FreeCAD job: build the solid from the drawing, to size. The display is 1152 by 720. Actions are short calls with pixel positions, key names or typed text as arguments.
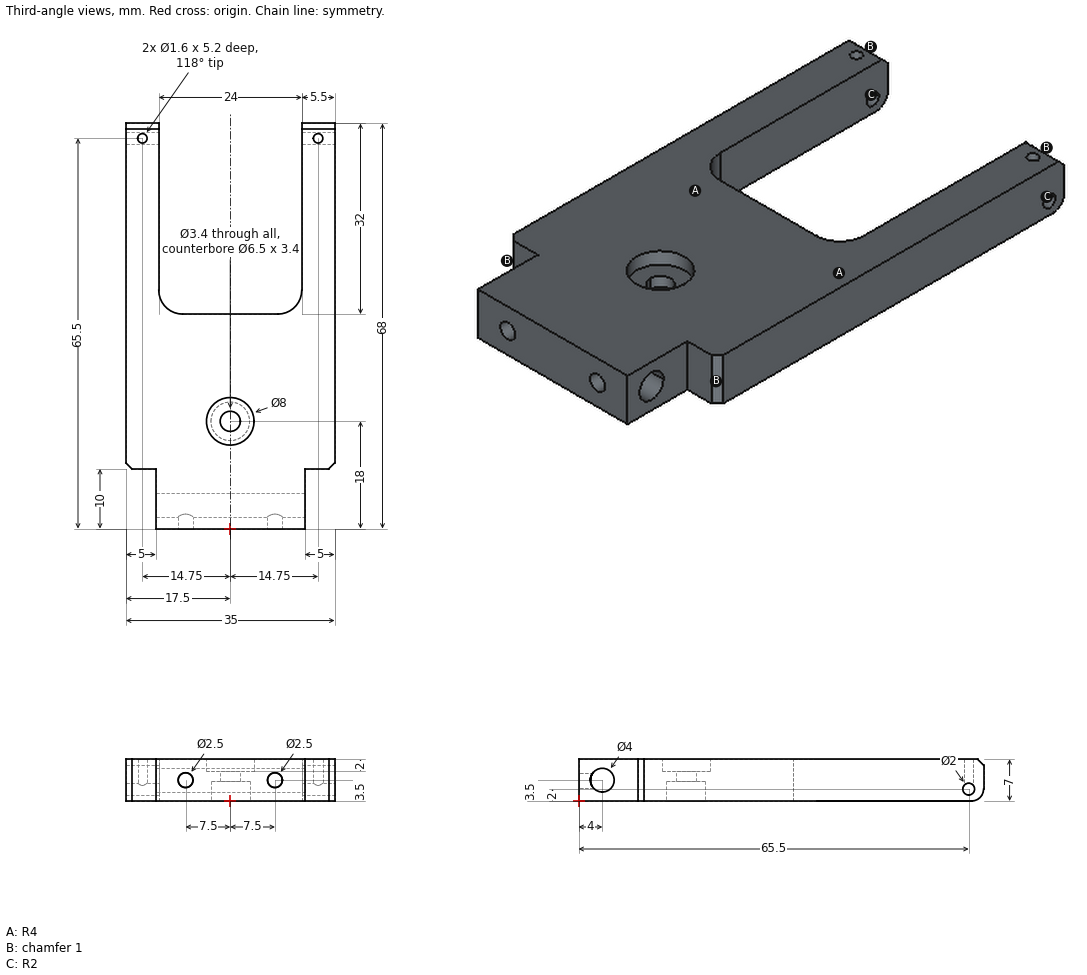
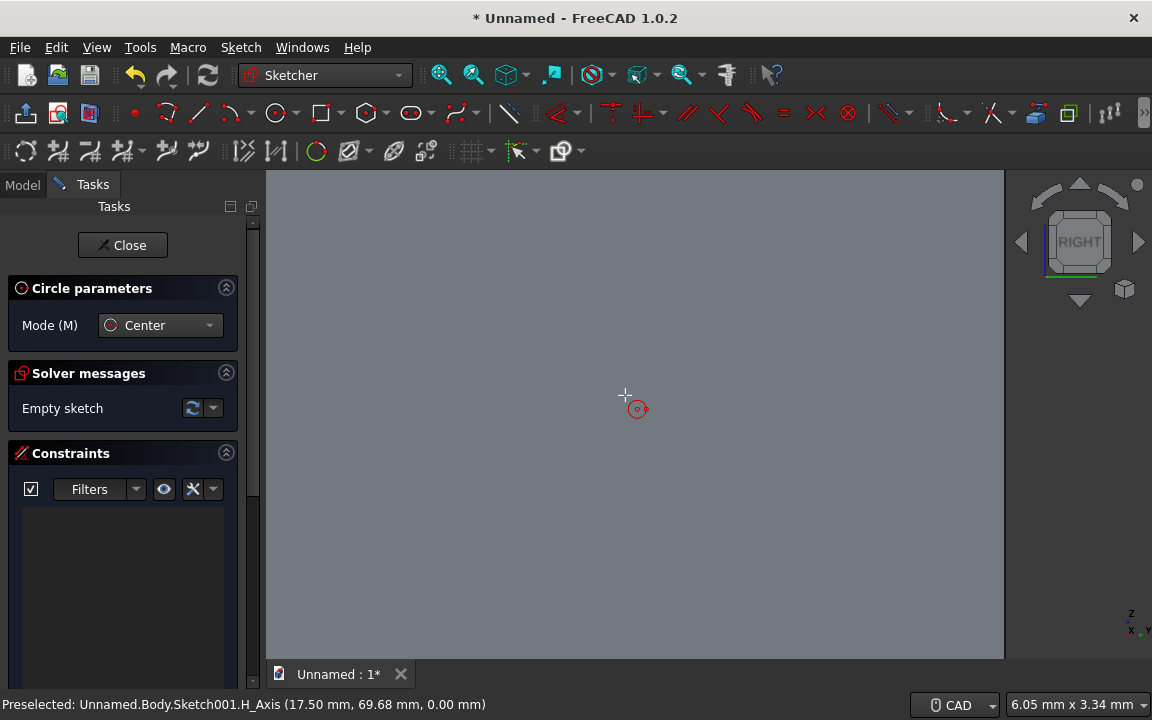
click(639, 412)
move(742, 309)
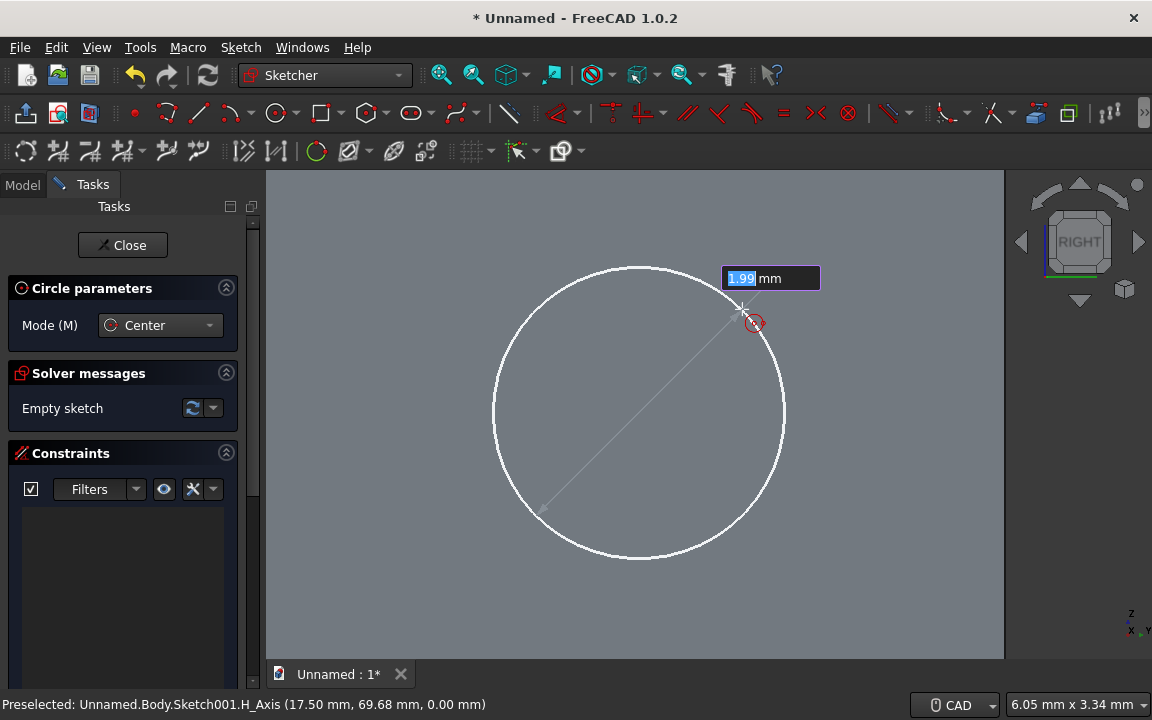
text(2)
key(Return)
key(Escape)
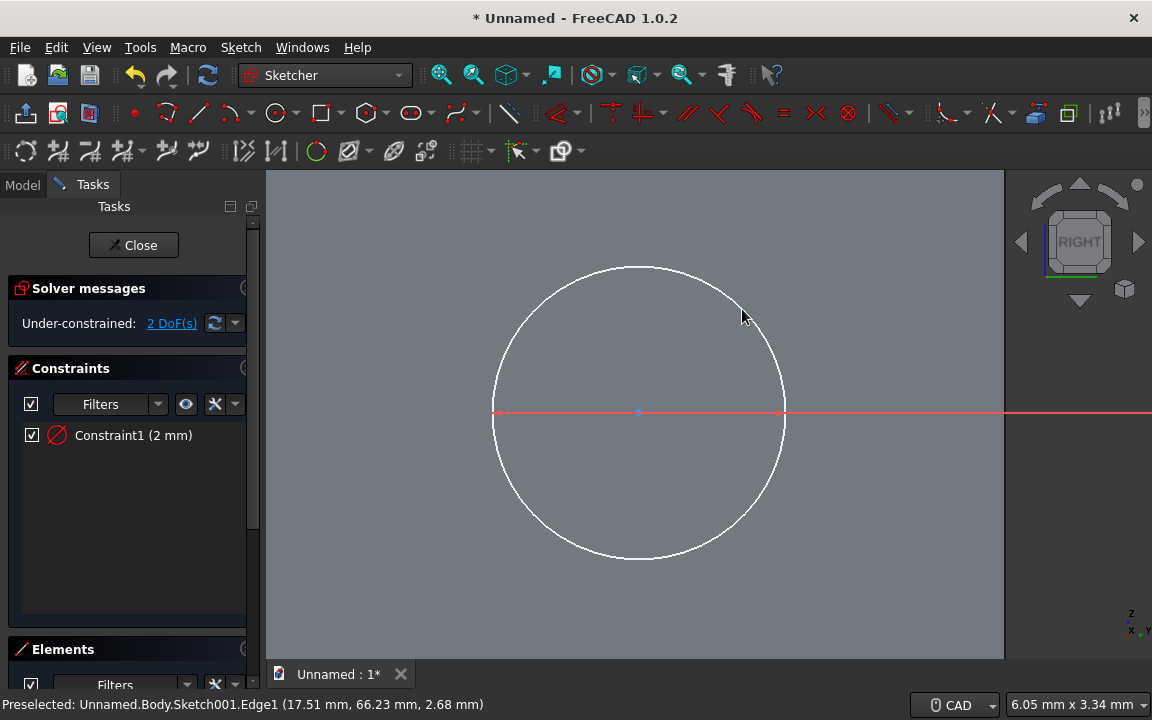
key(d)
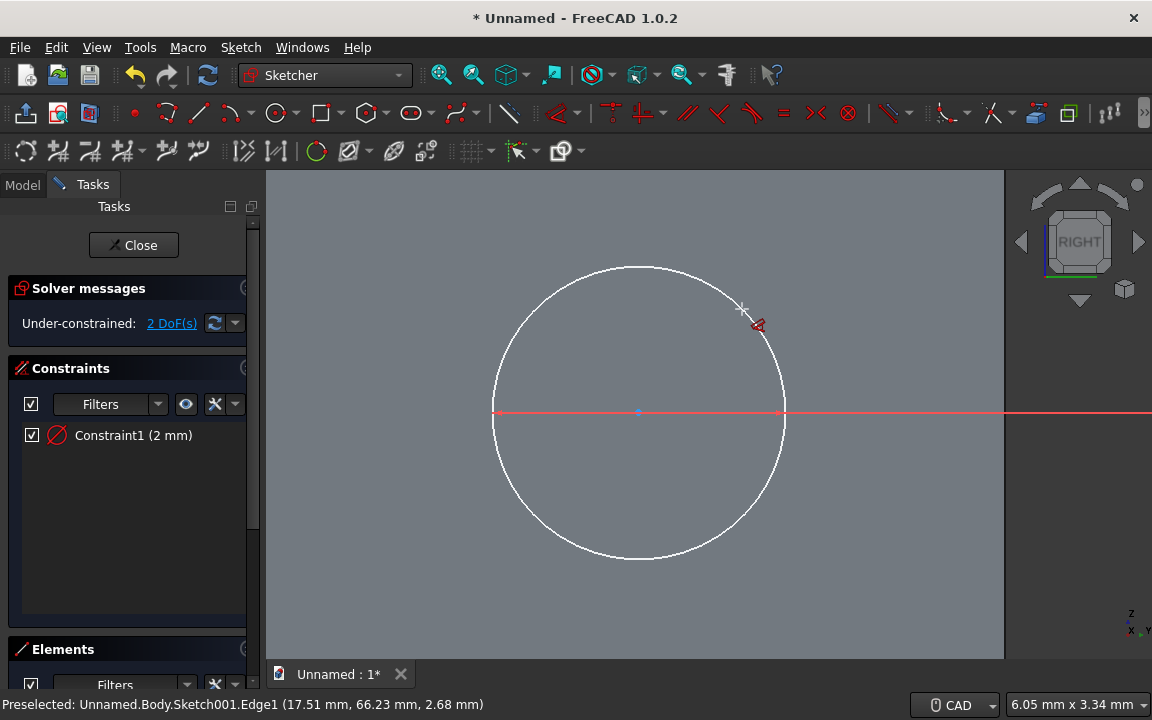
click(639, 413)
click(673, 522)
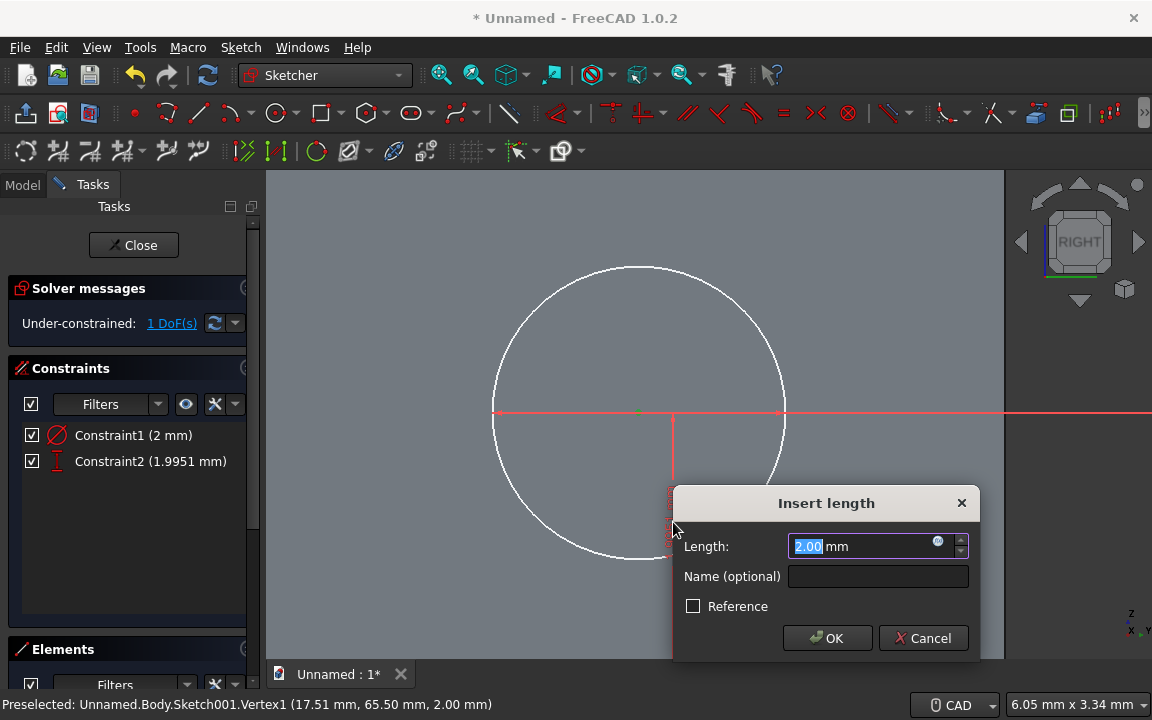
text(2)
key(Return)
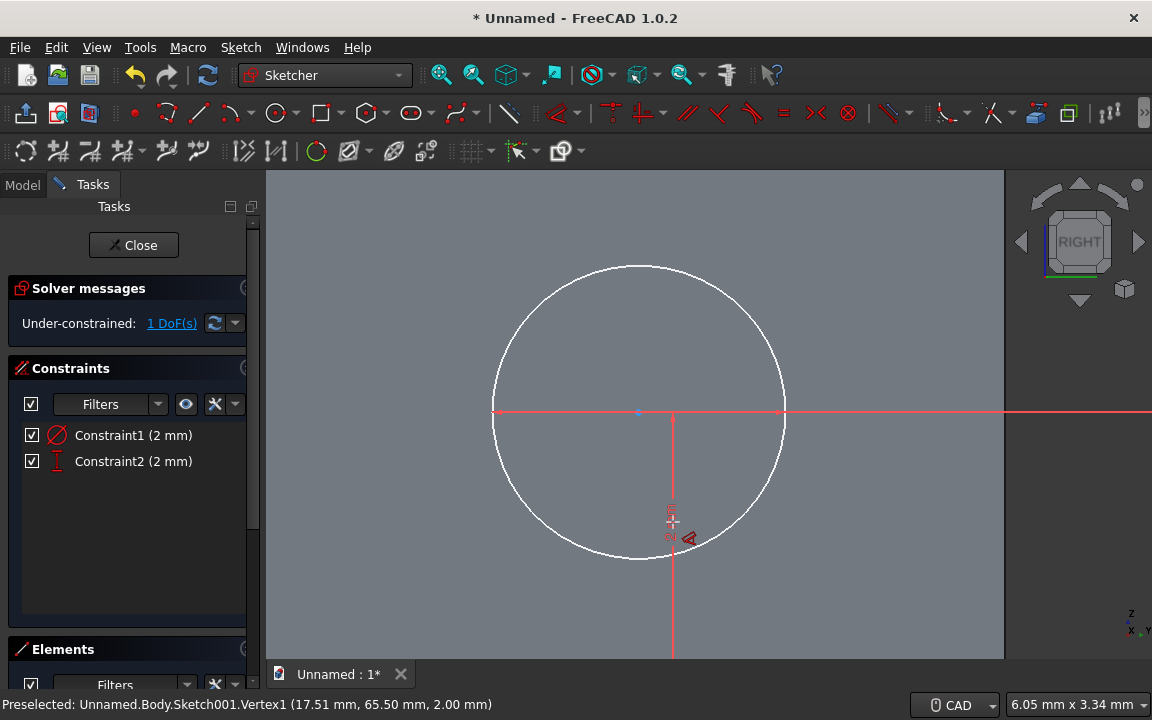
click(639, 412)
click(466, 378)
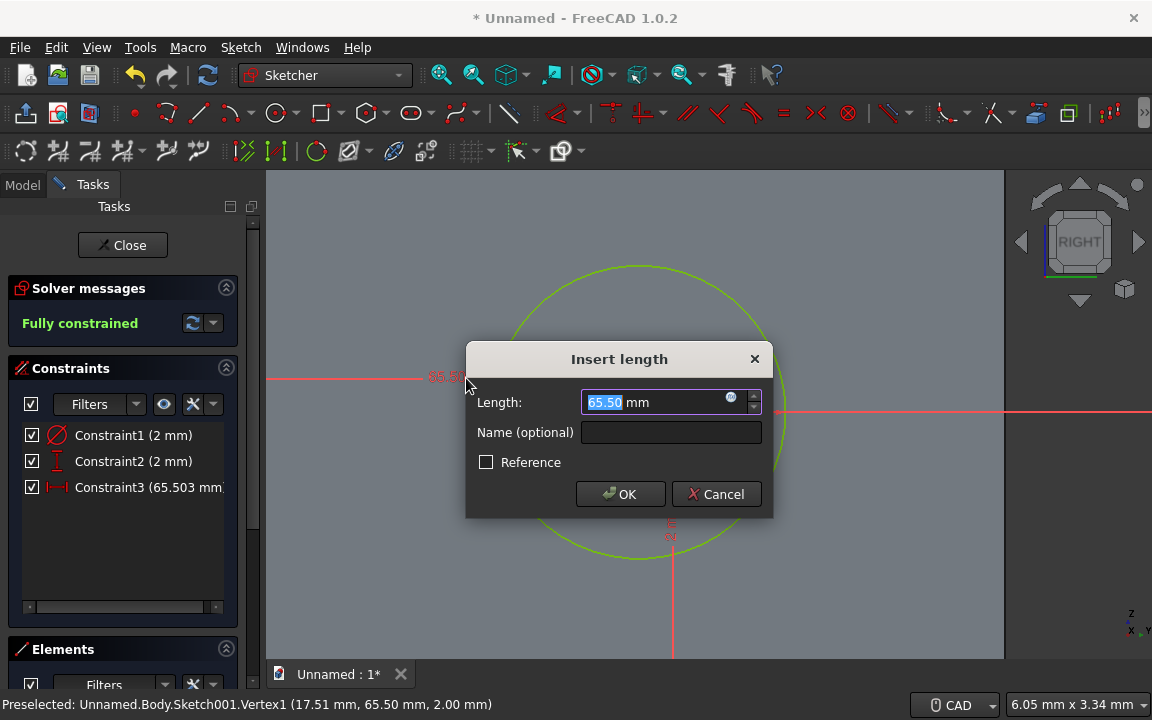
text(65.5)
key(Return)
key(Escape)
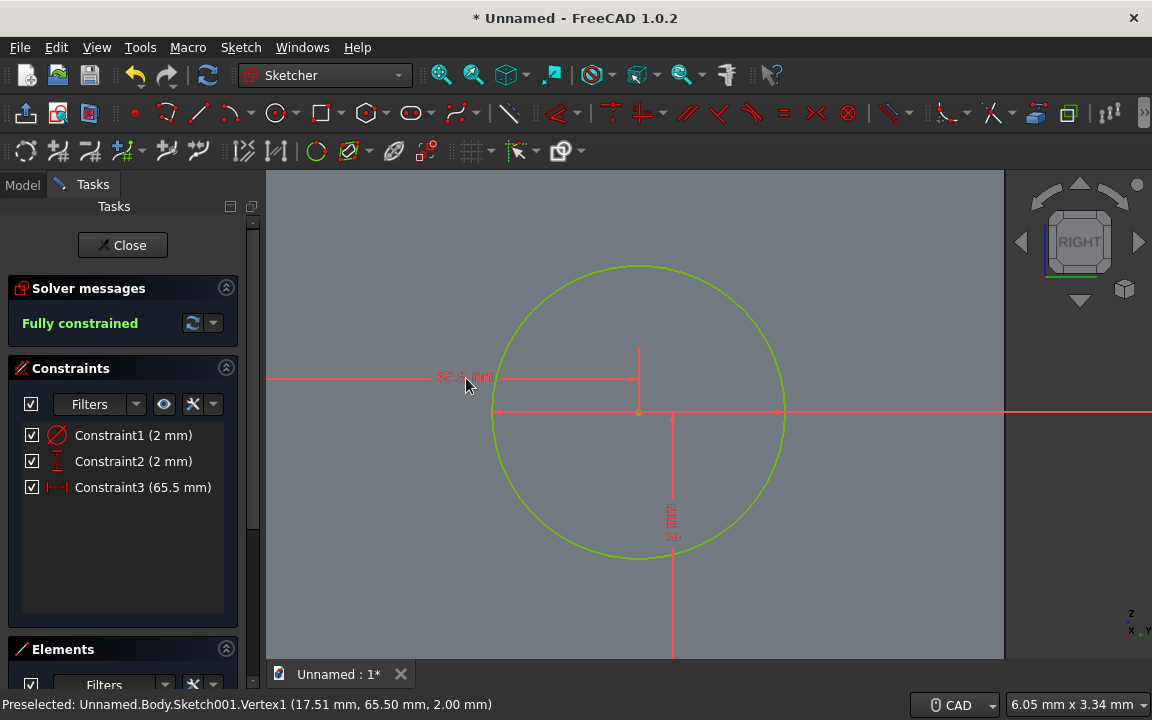
click(123, 245)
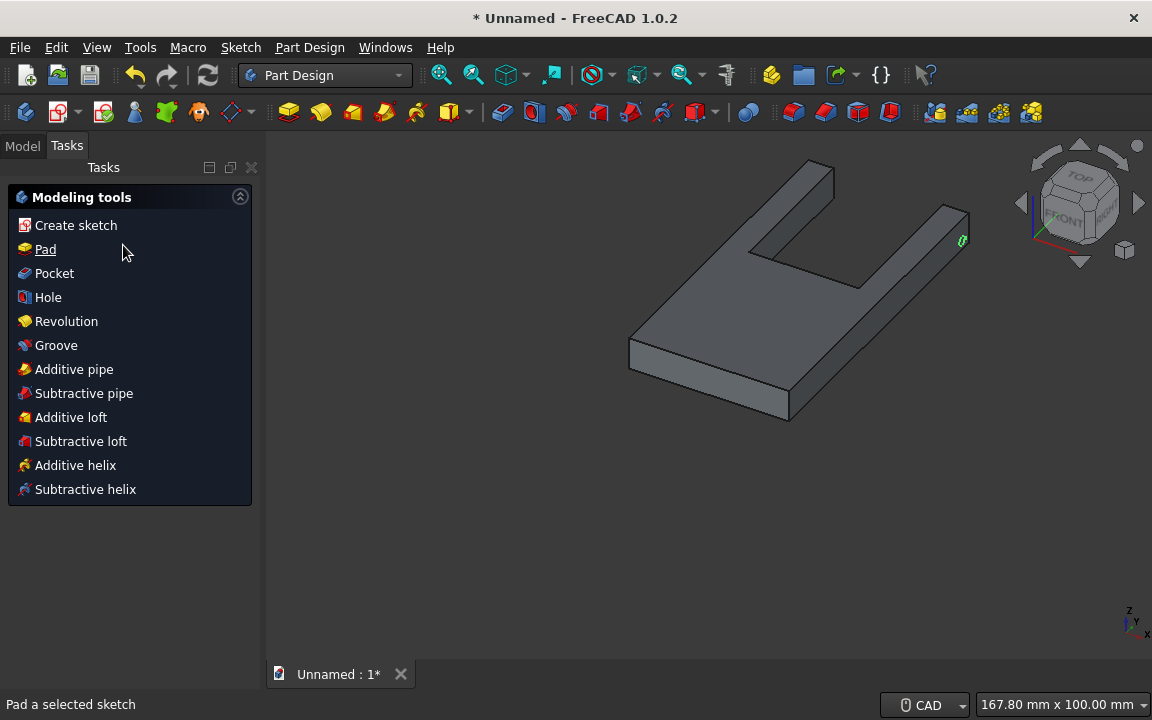
click(504, 112)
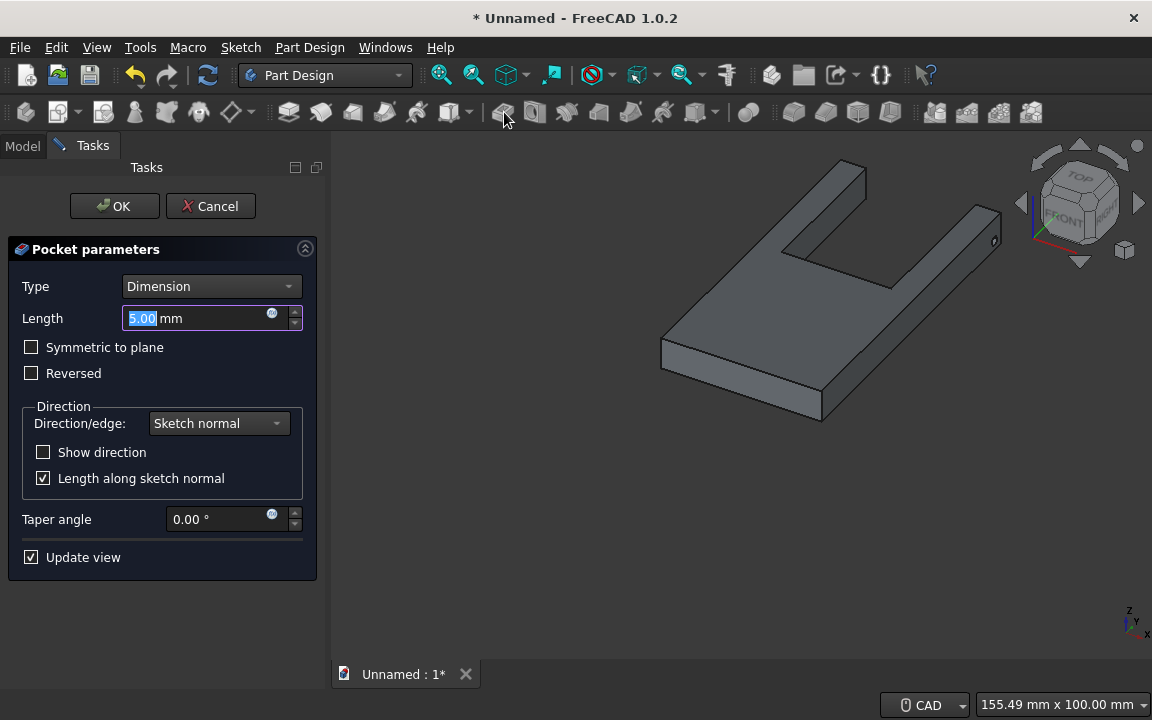
click(212, 286)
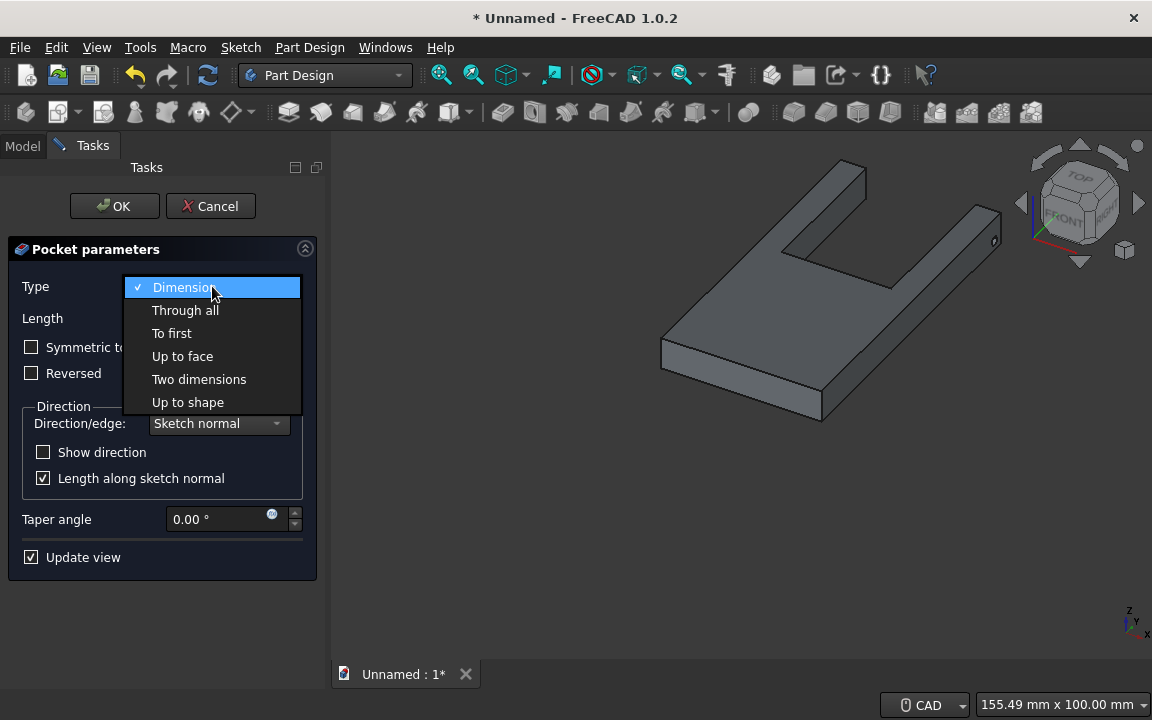
click(212, 310)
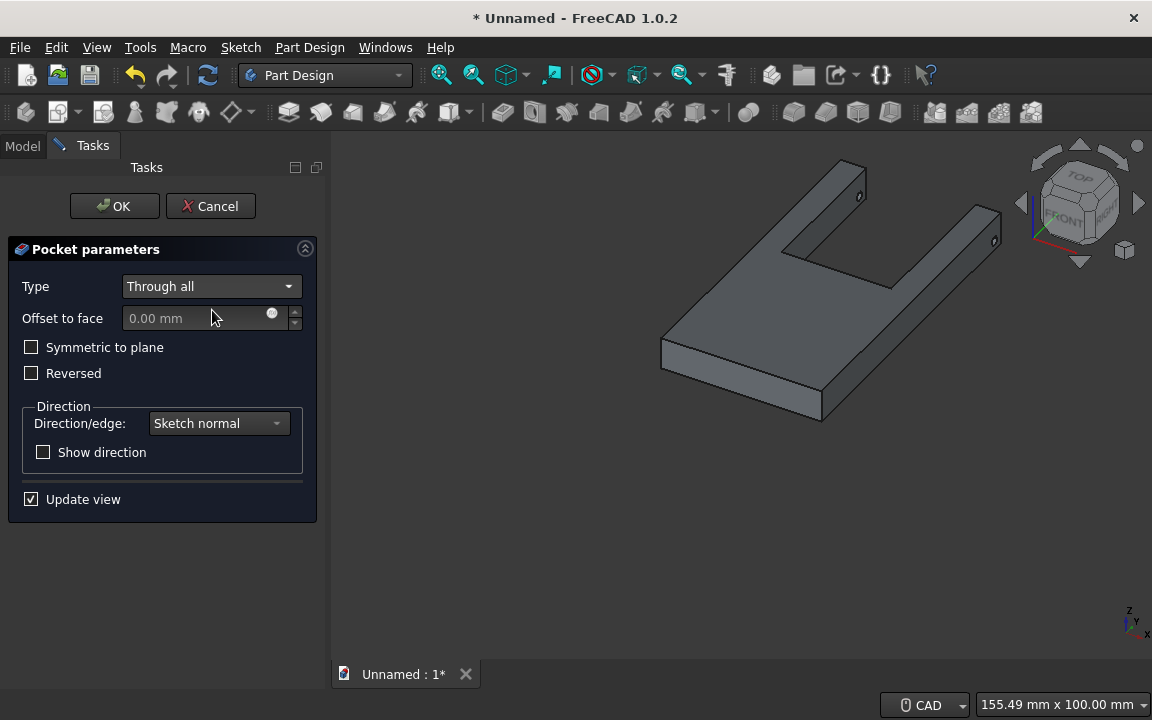
click(115, 206)